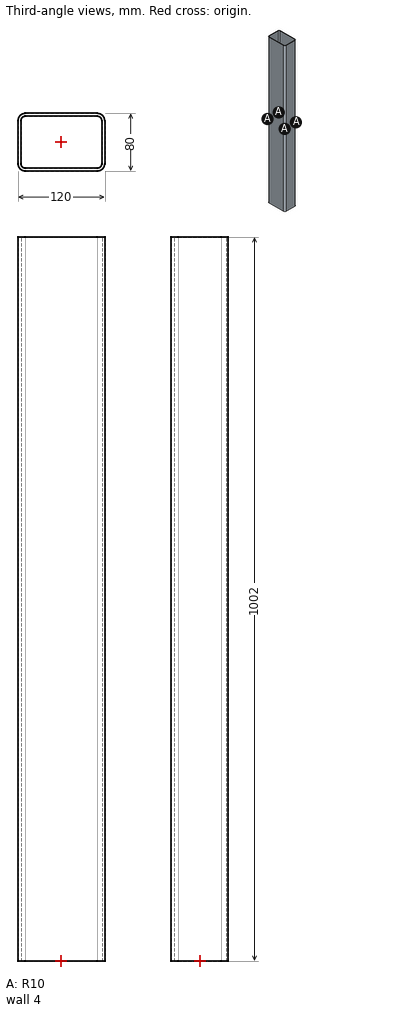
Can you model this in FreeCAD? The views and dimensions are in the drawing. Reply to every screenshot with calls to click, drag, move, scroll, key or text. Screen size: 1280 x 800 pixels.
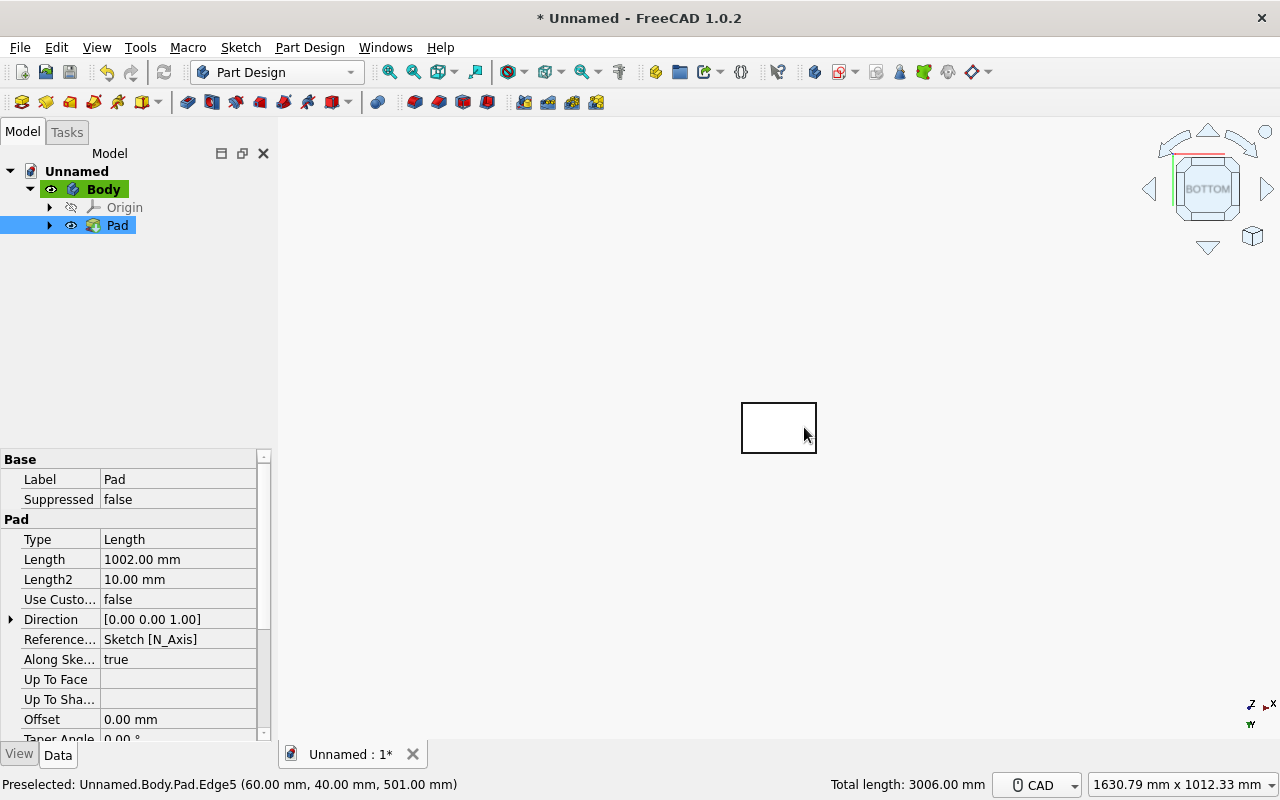
click(390, 72)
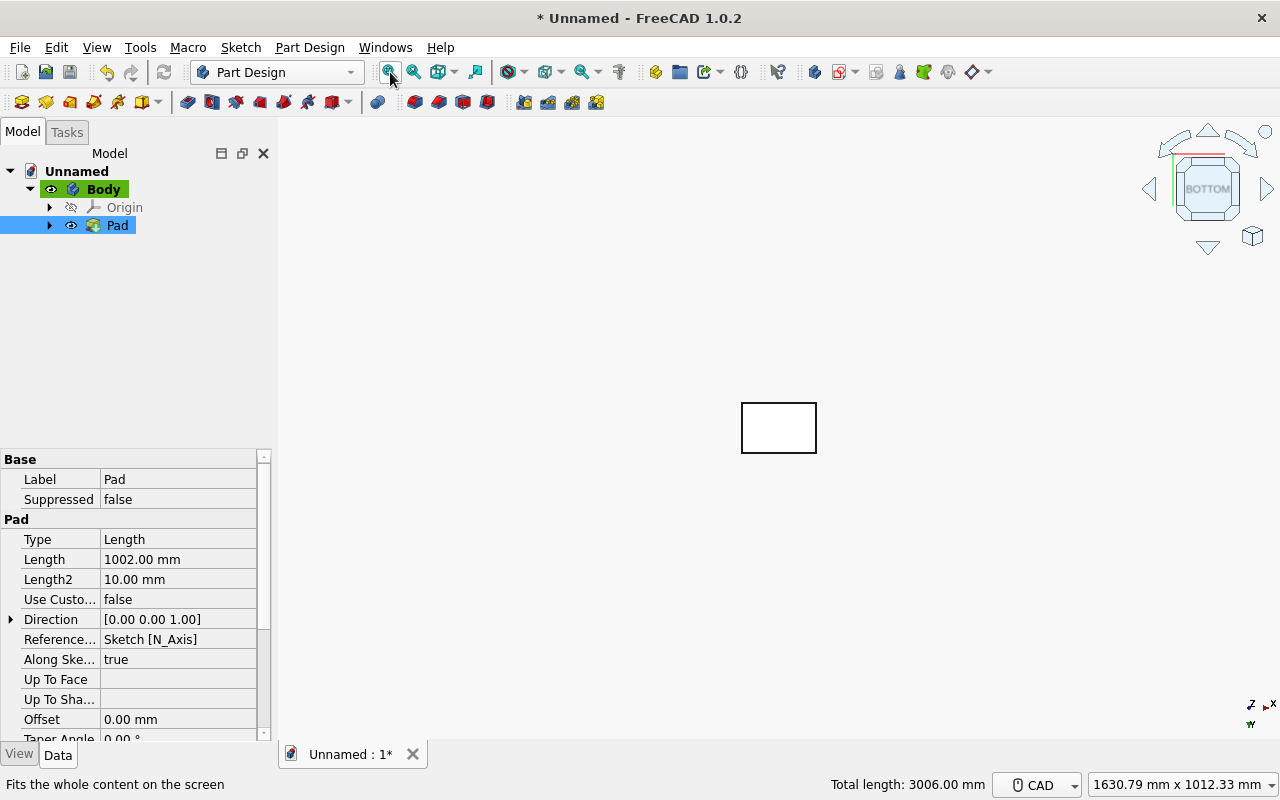
key(4)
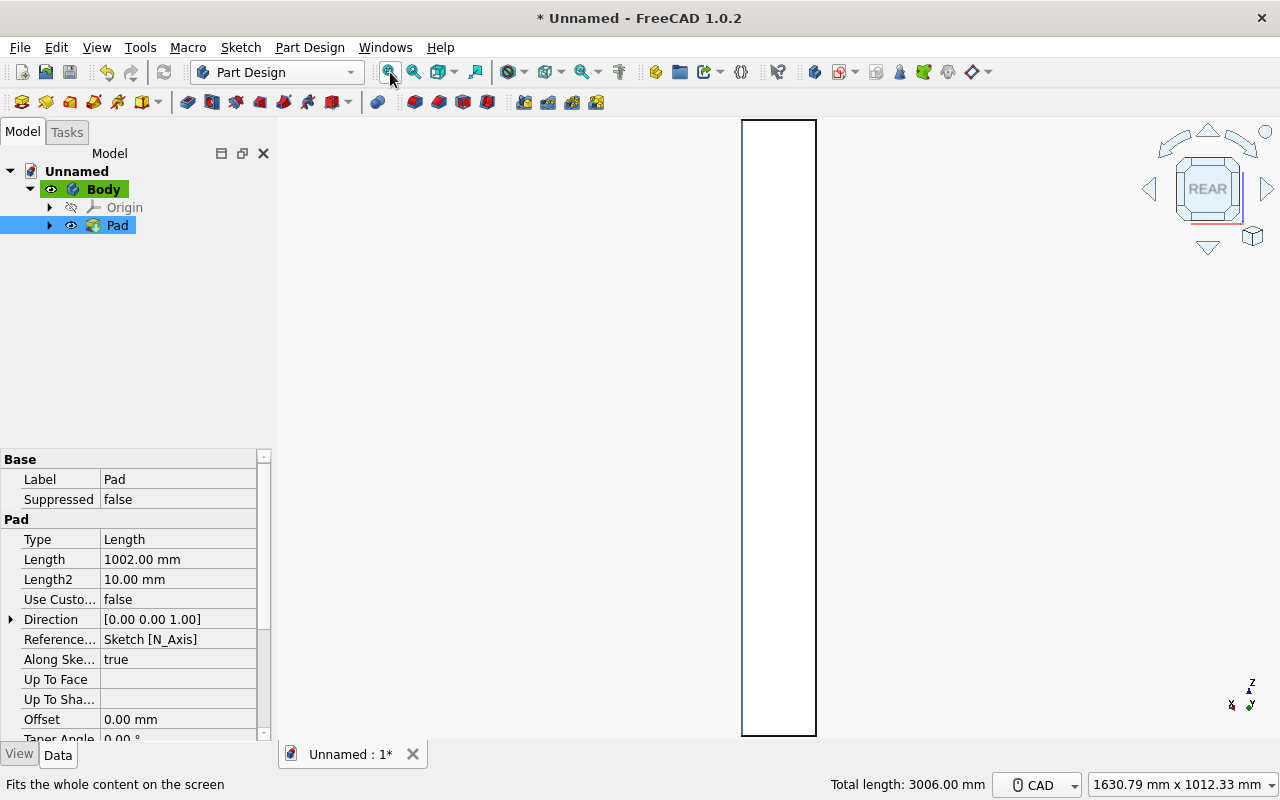
click(816, 427, ctrl)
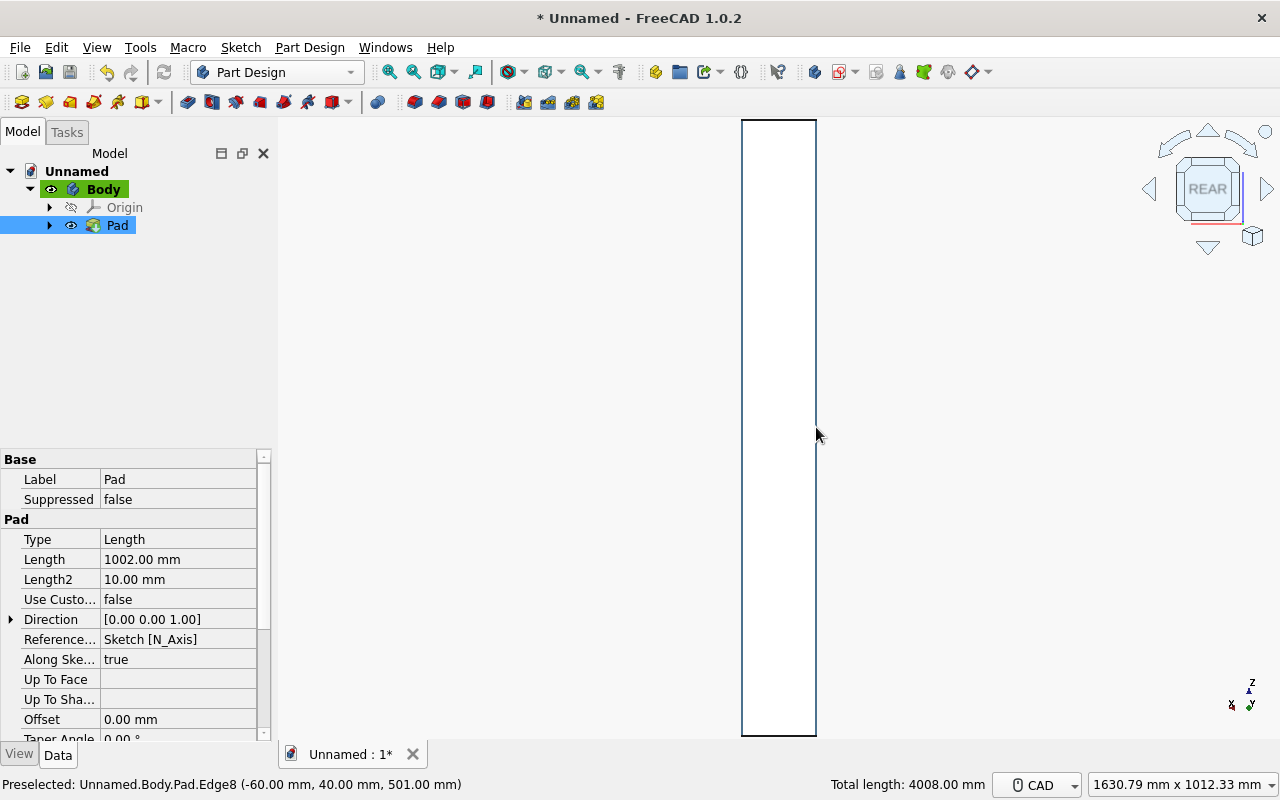
click(416, 102)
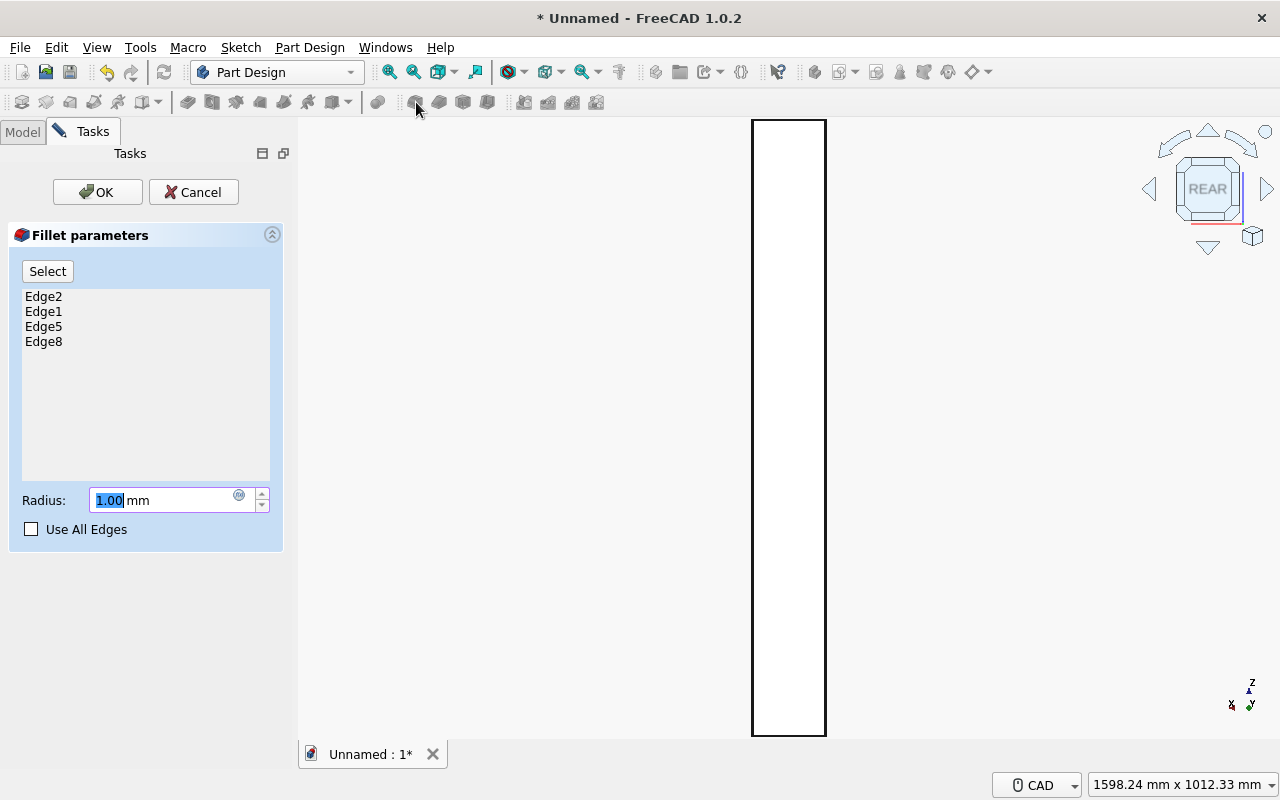
text(10)
key(Tab)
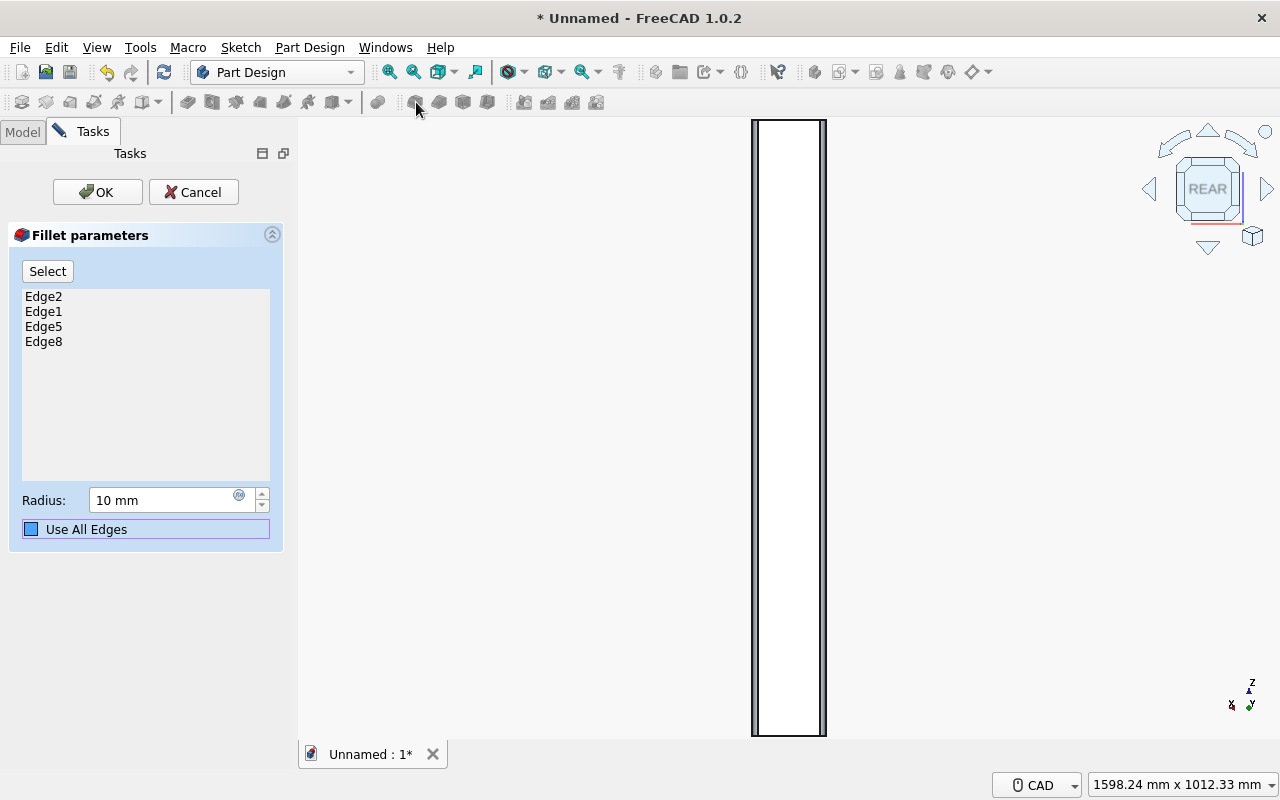
click(98, 192)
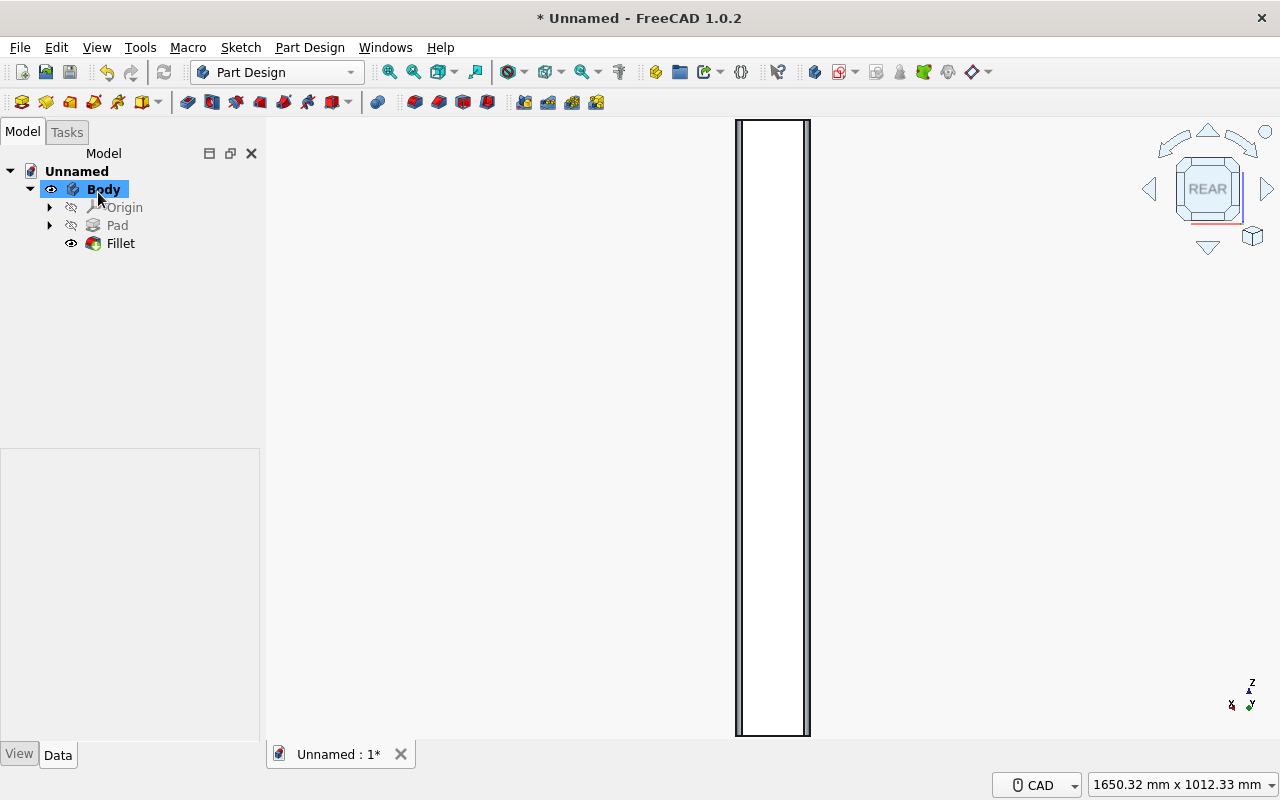
key(0)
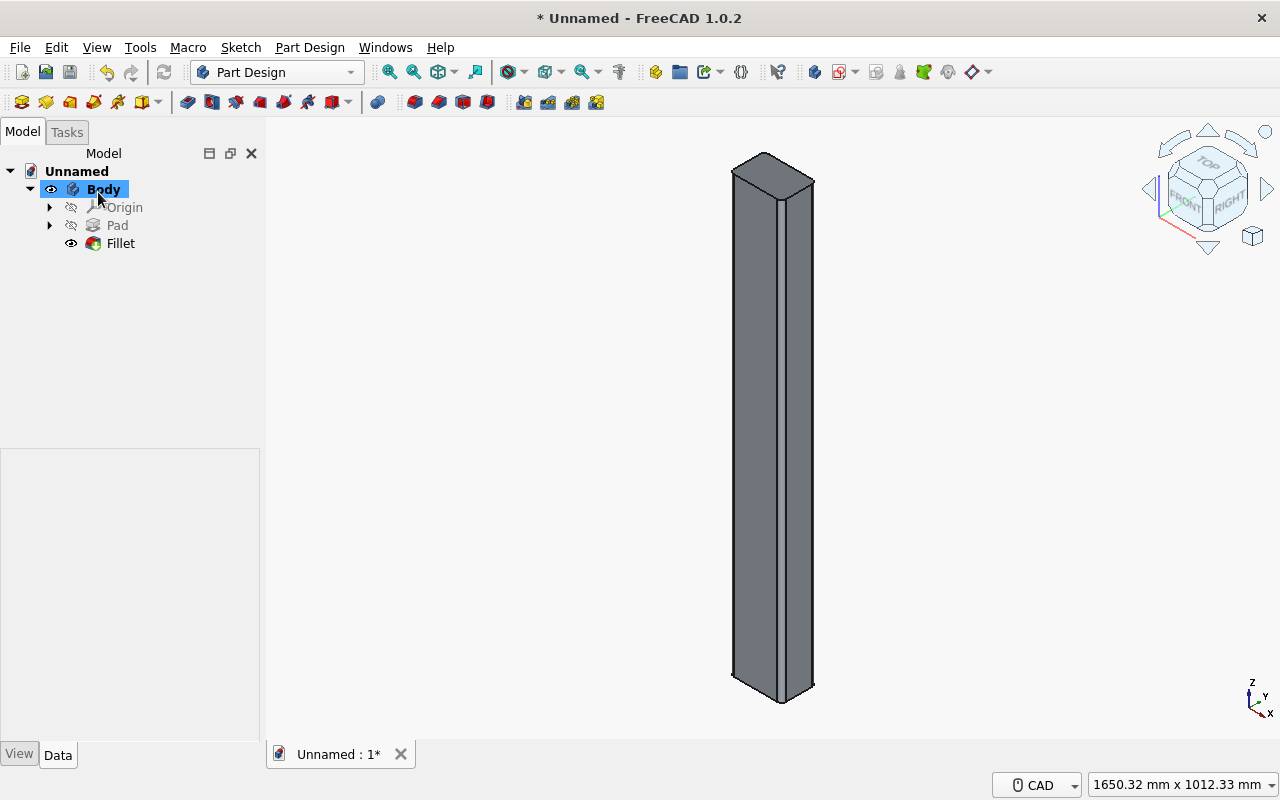
click(780, 180)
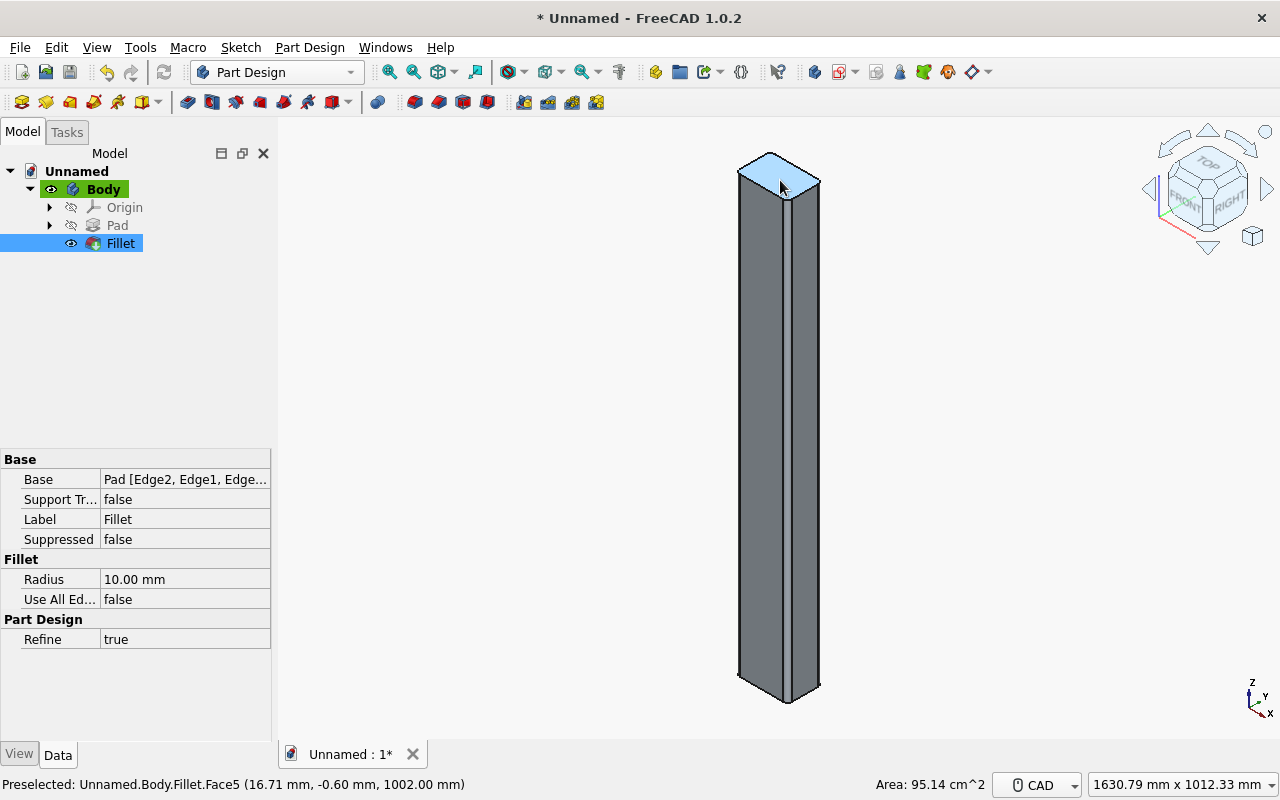
key(2)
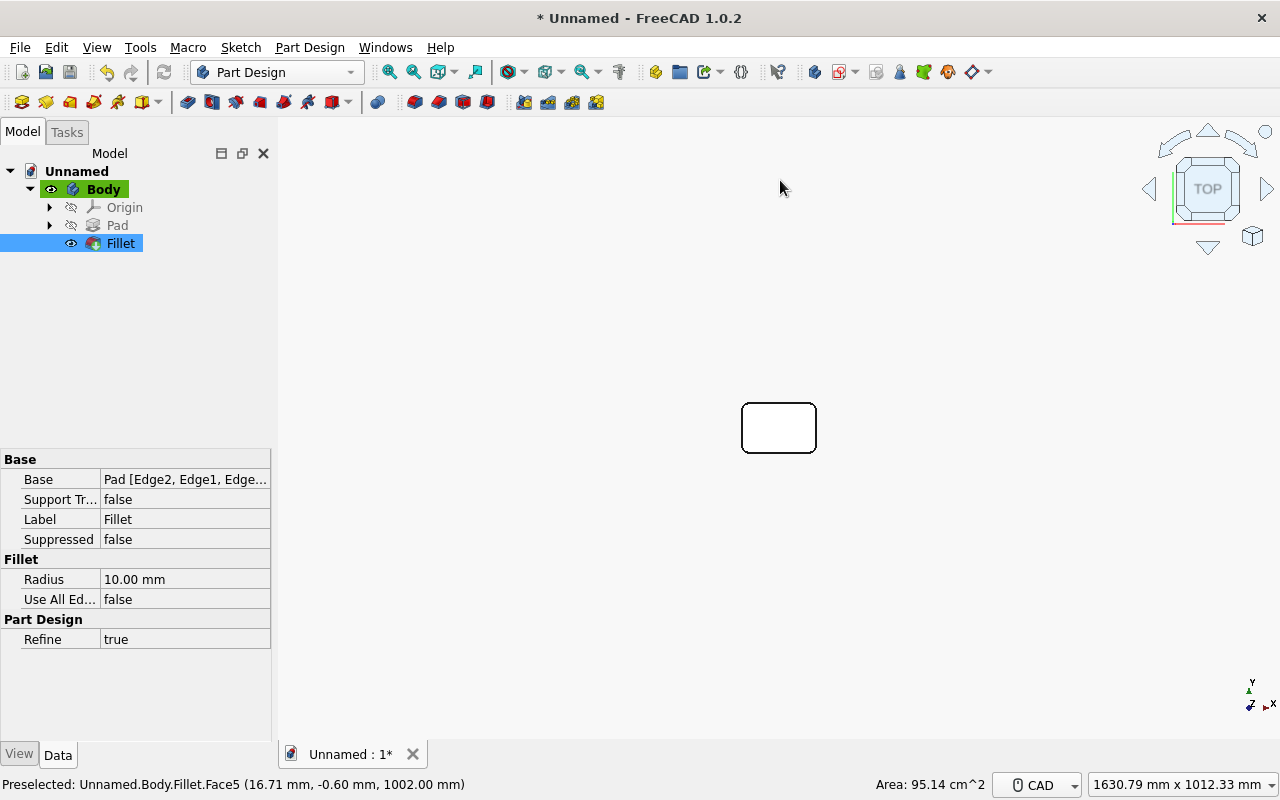
click(390, 72)